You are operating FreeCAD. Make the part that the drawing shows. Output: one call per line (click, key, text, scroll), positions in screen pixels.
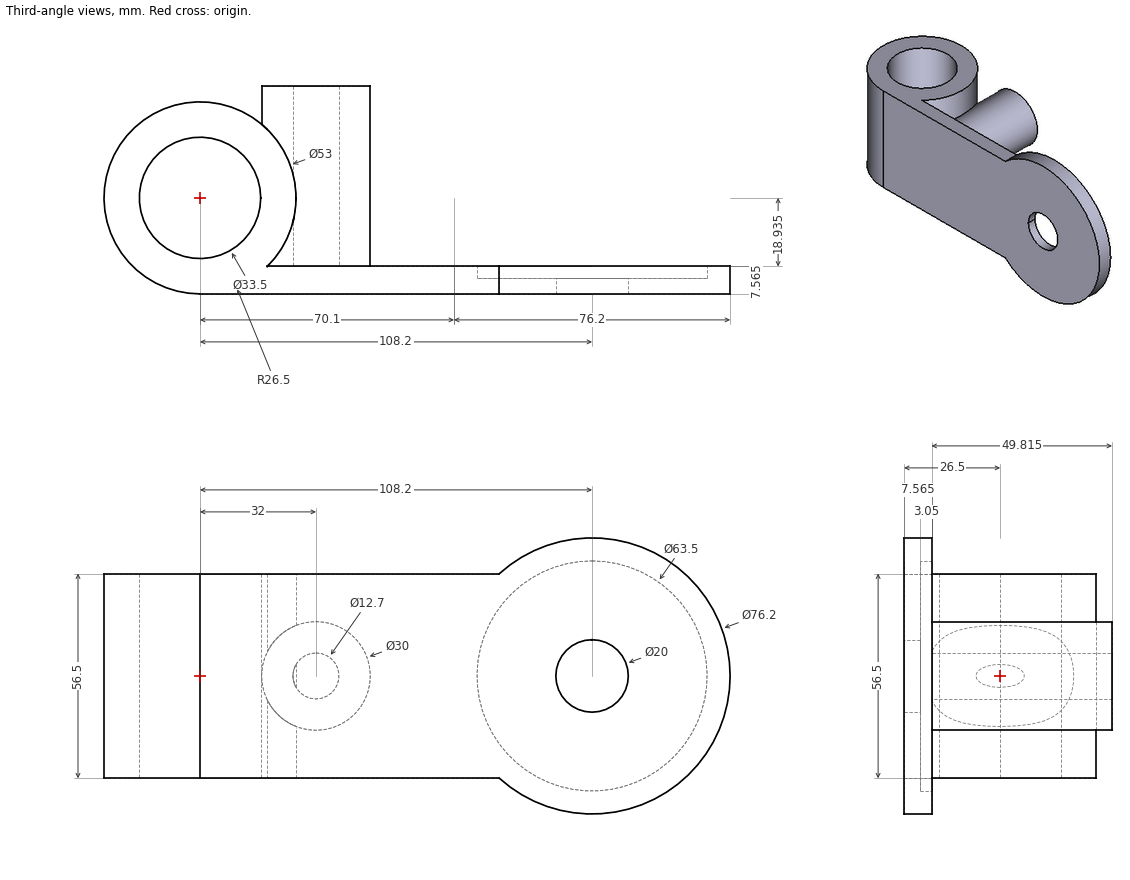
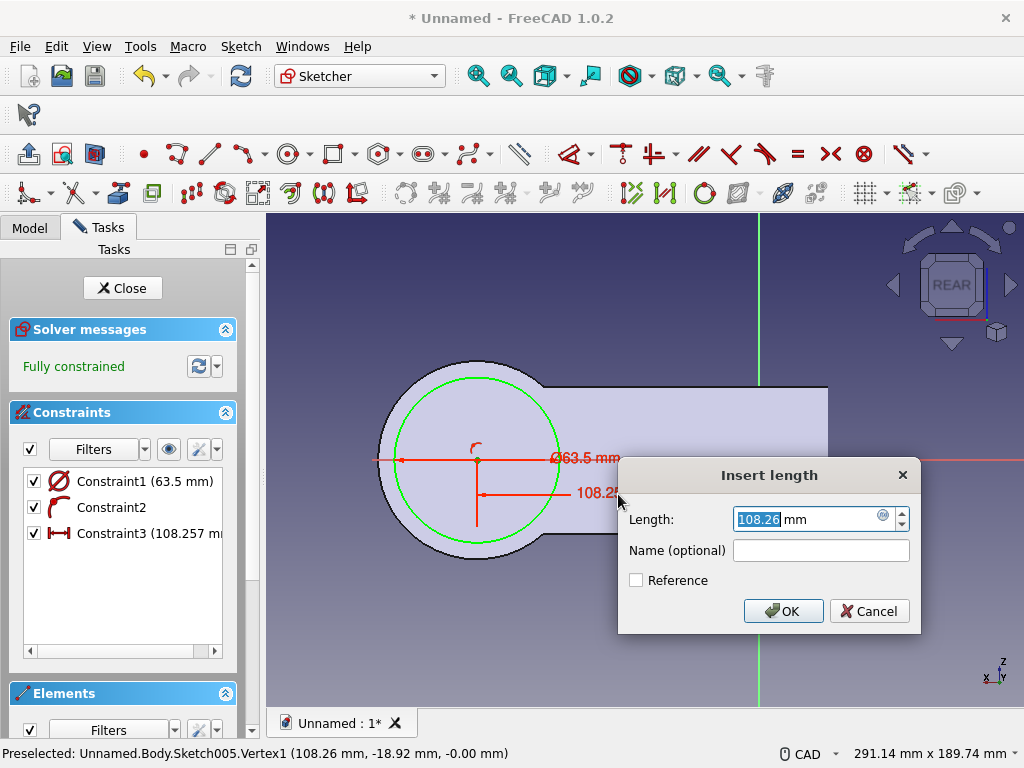
text(108.2)
key(Return)
key(Escape)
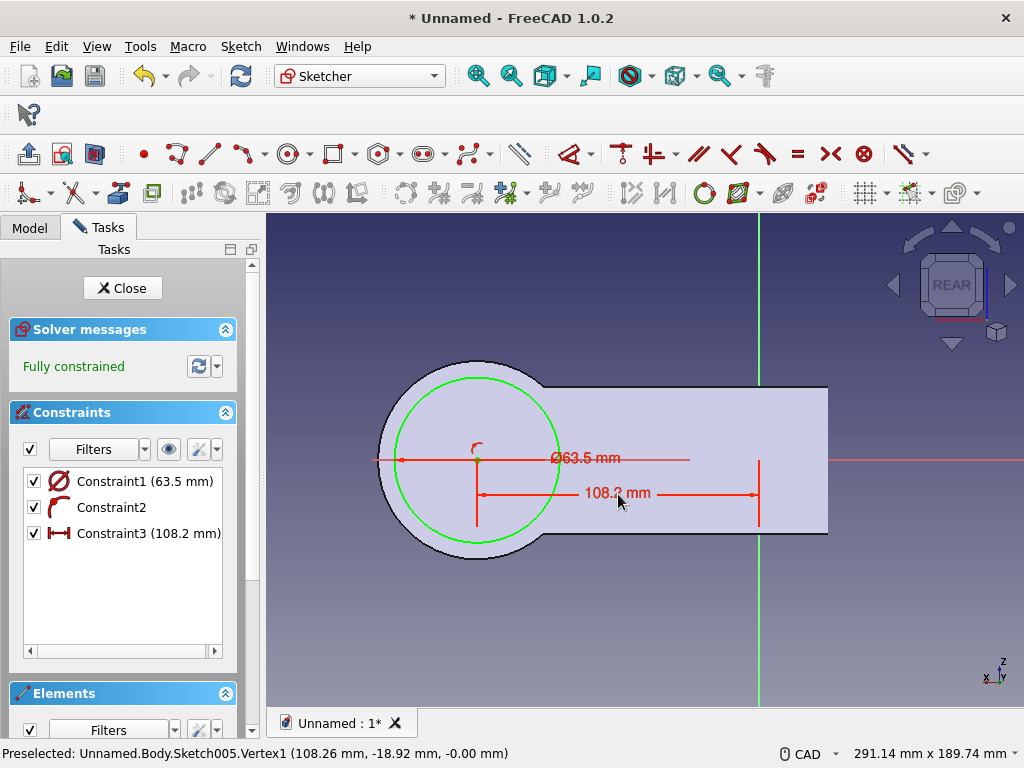
click(123, 288)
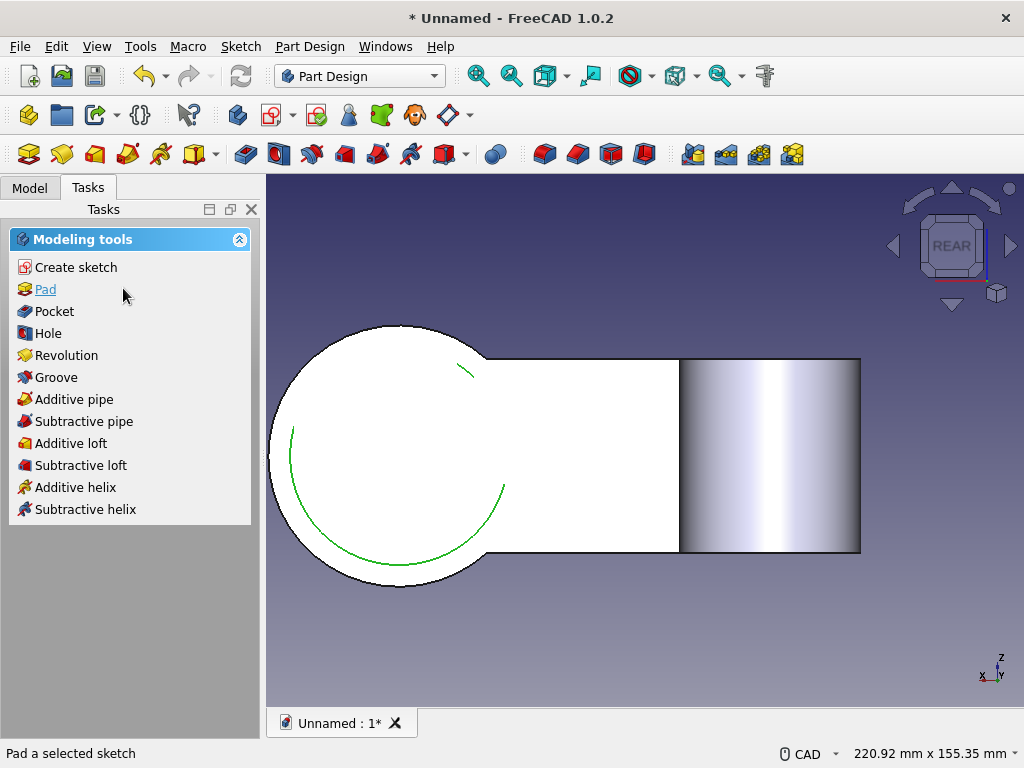
click(246, 154)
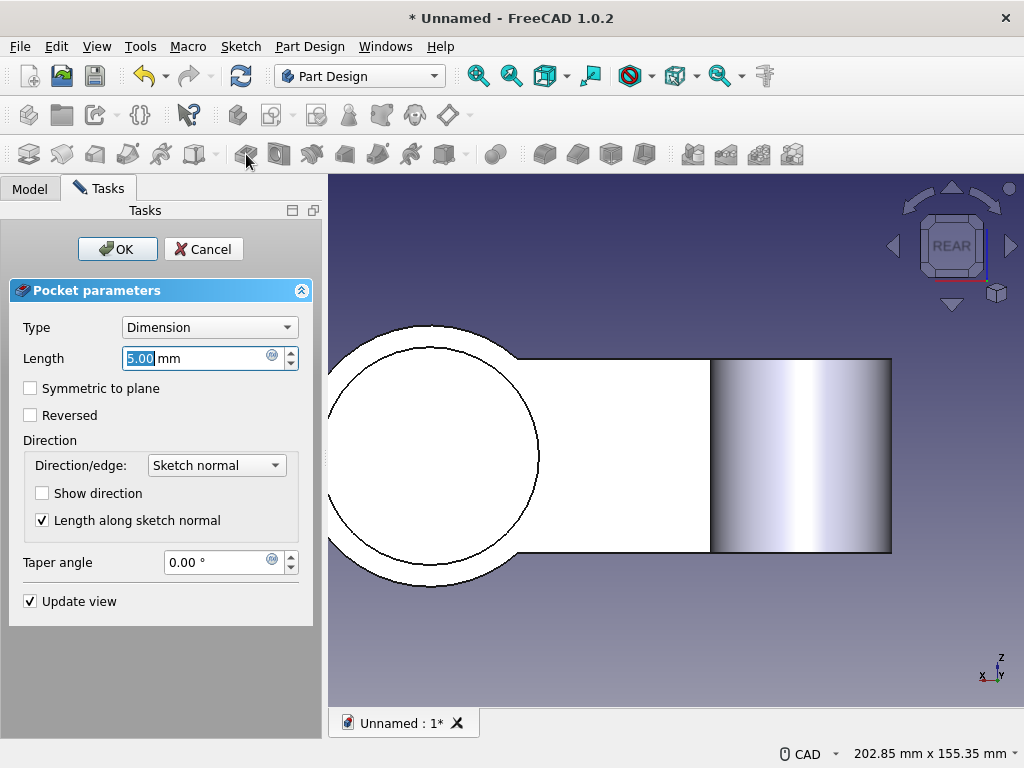
text(3.05)
key(Tab)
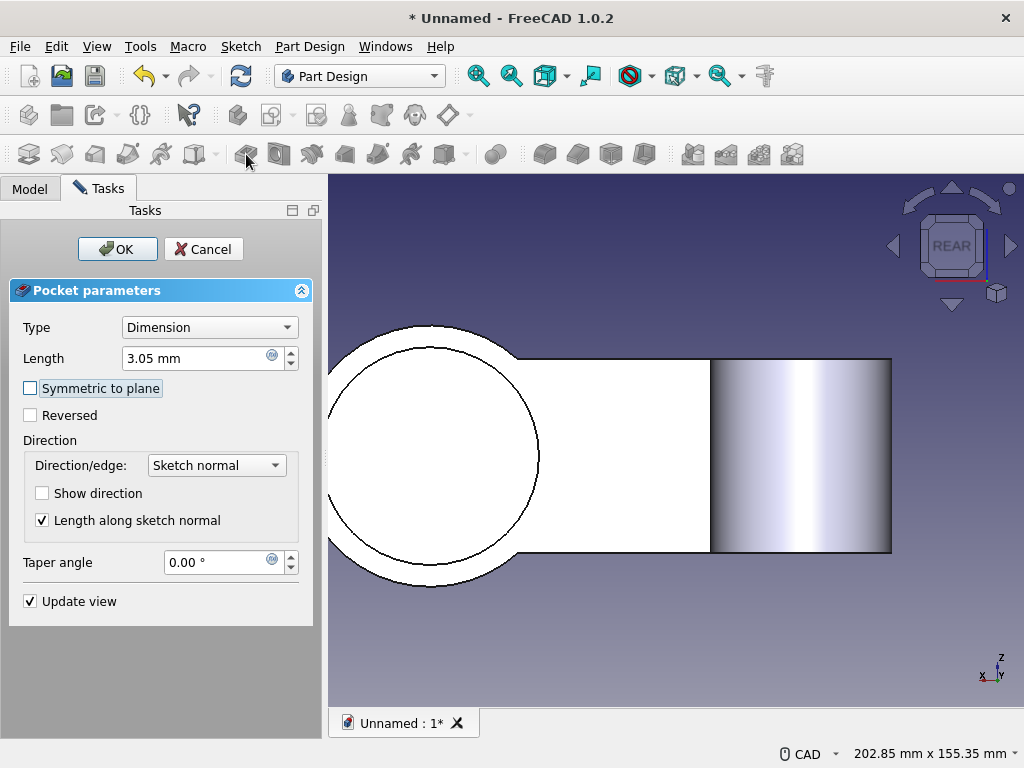
click(118, 249)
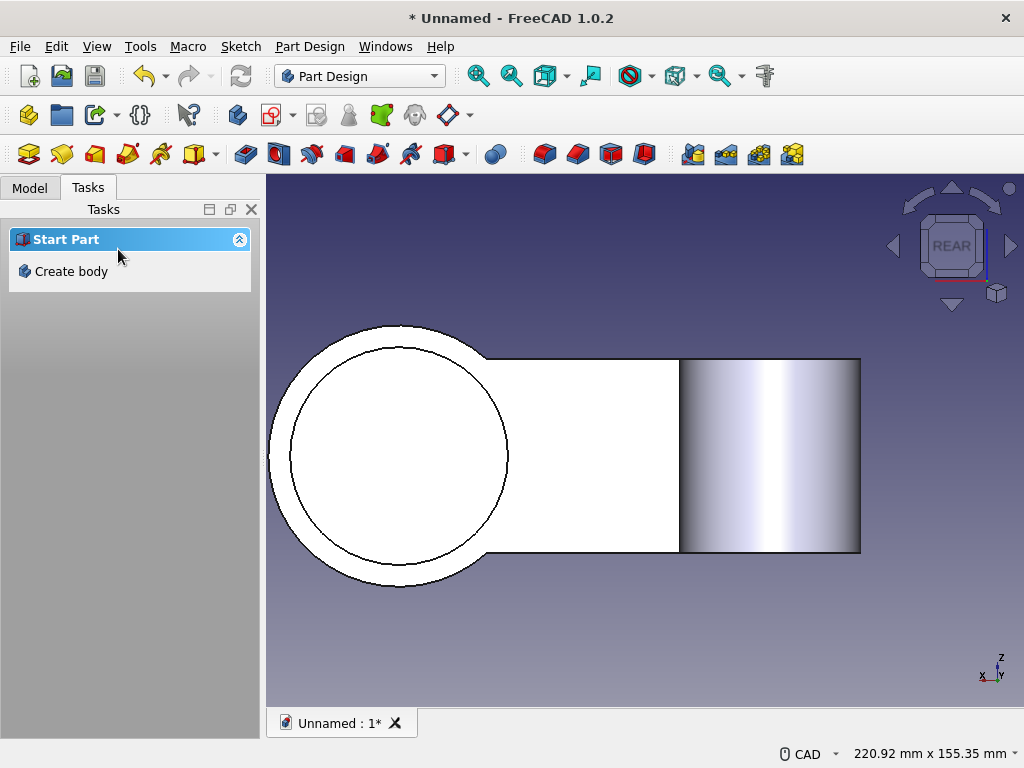
click(399, 455)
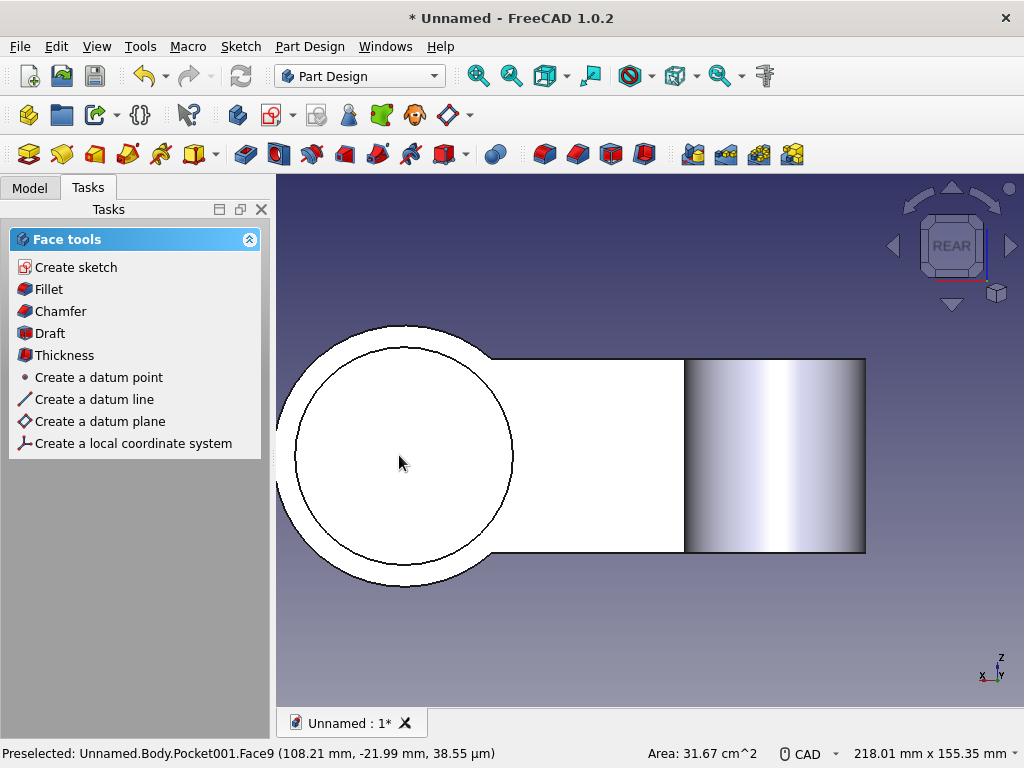
click(270, 116)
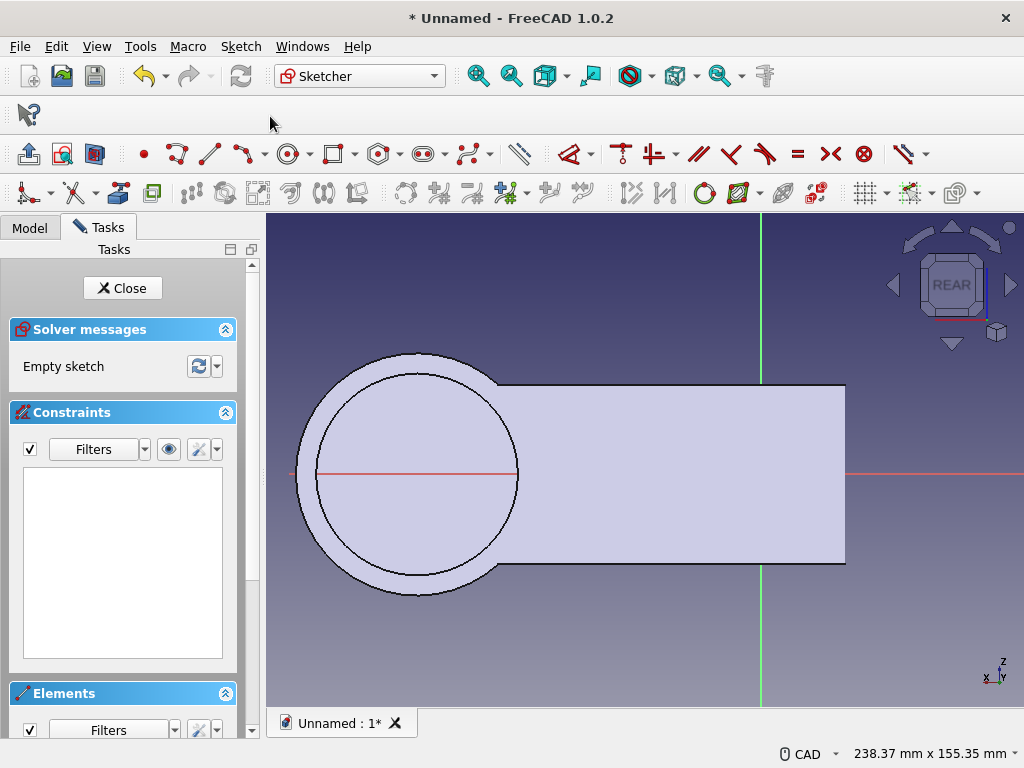
scroll(377, 478, up, 8)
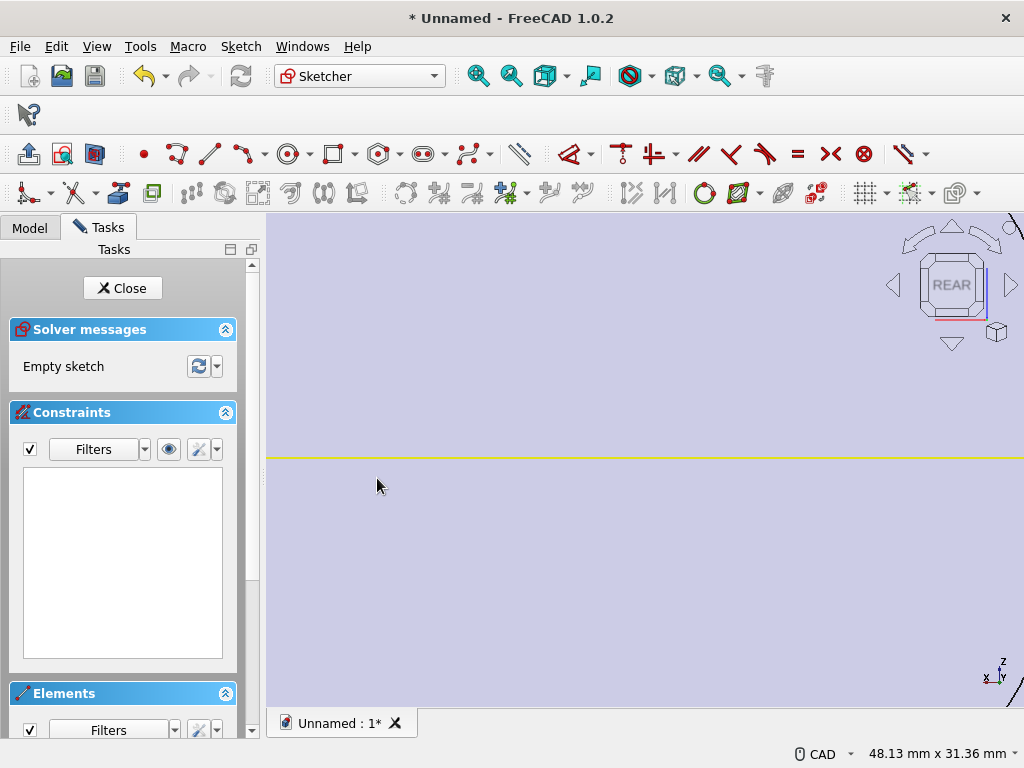
key(g)
key(c)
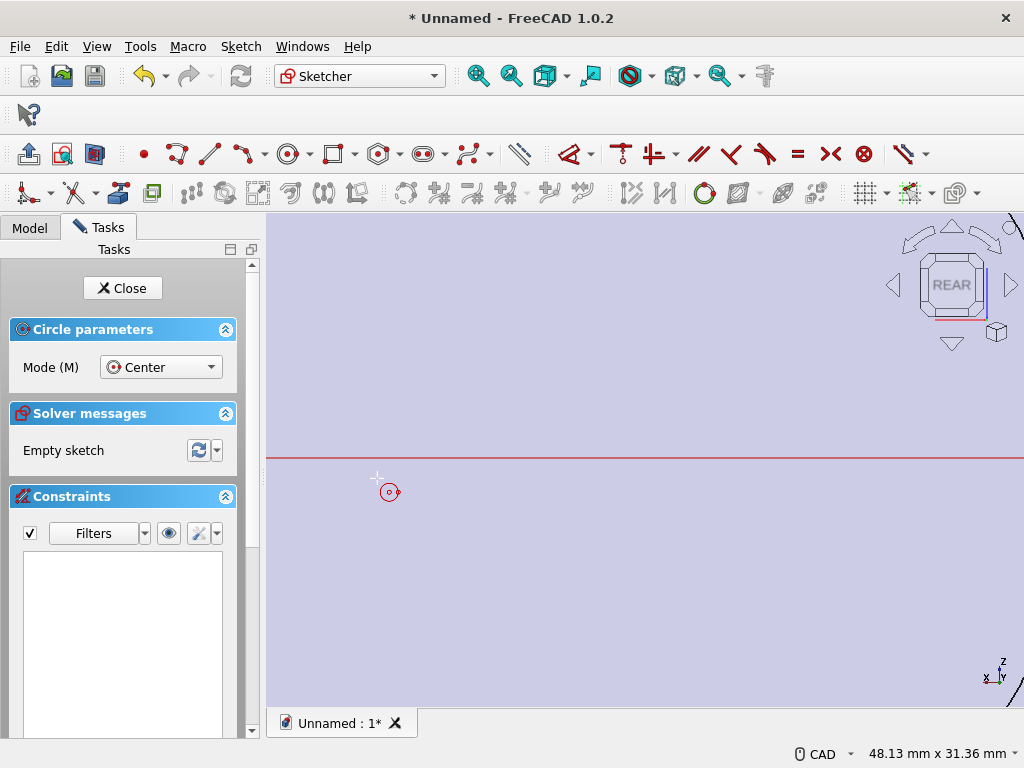
click(575, 458)
move(686, 347)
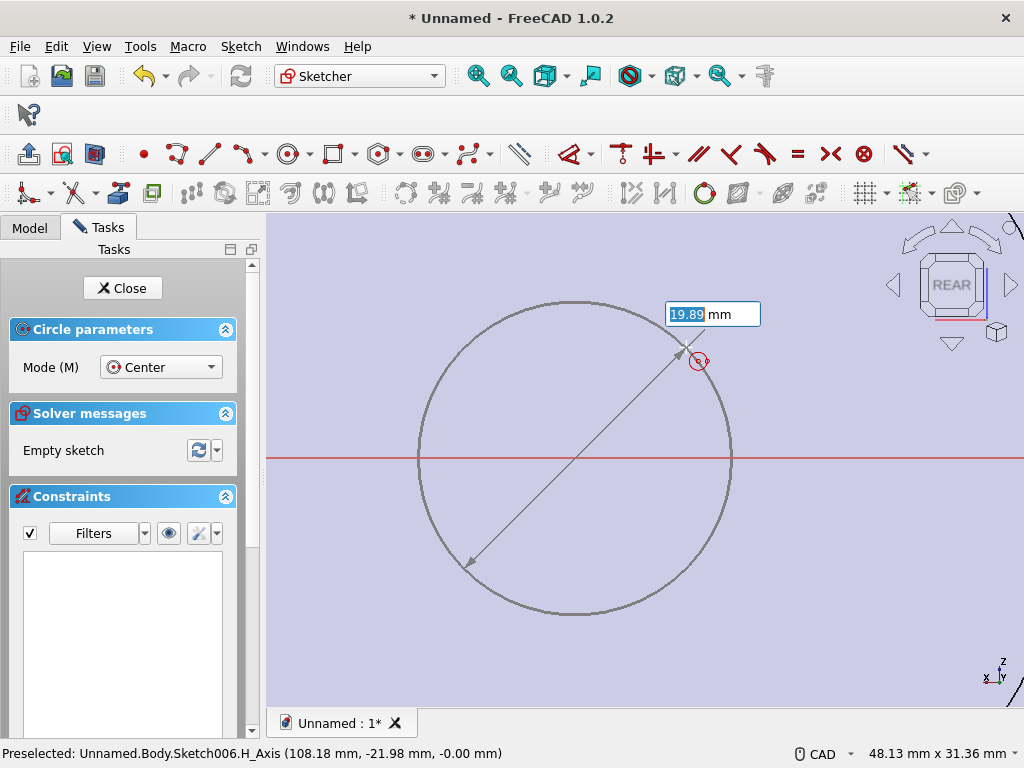
text(20)
key(Return)
key(Escape)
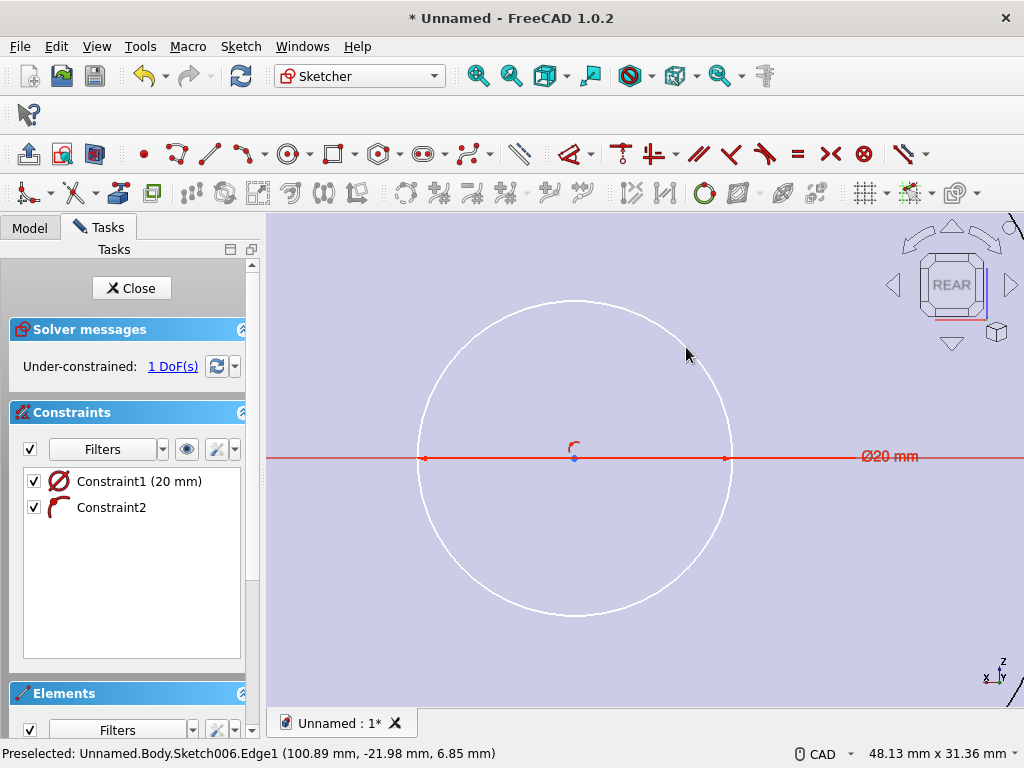
key(d)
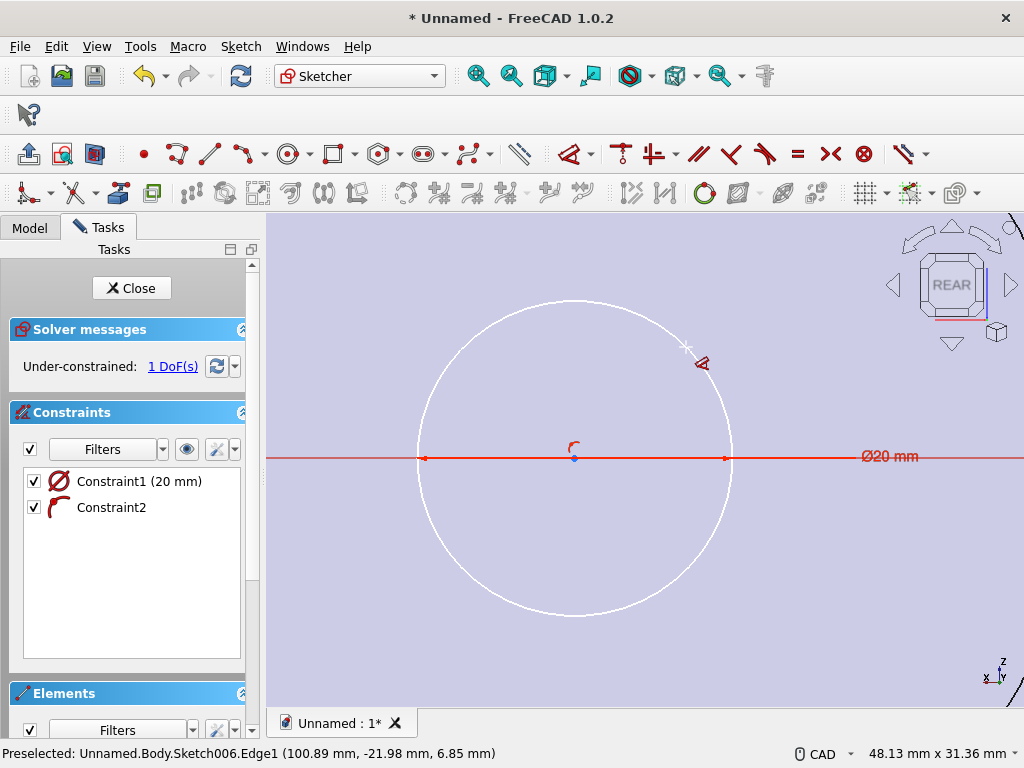
click(575, 458)
click(652, 492)